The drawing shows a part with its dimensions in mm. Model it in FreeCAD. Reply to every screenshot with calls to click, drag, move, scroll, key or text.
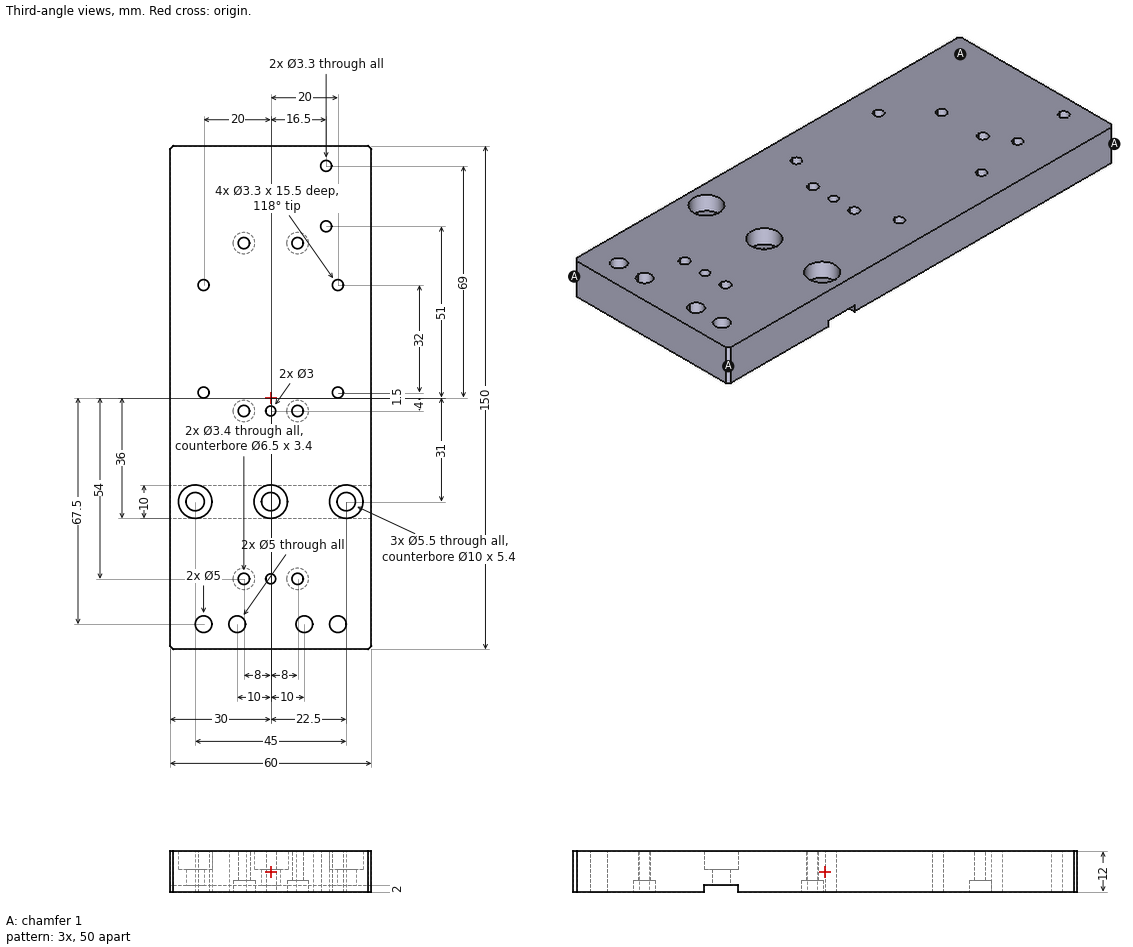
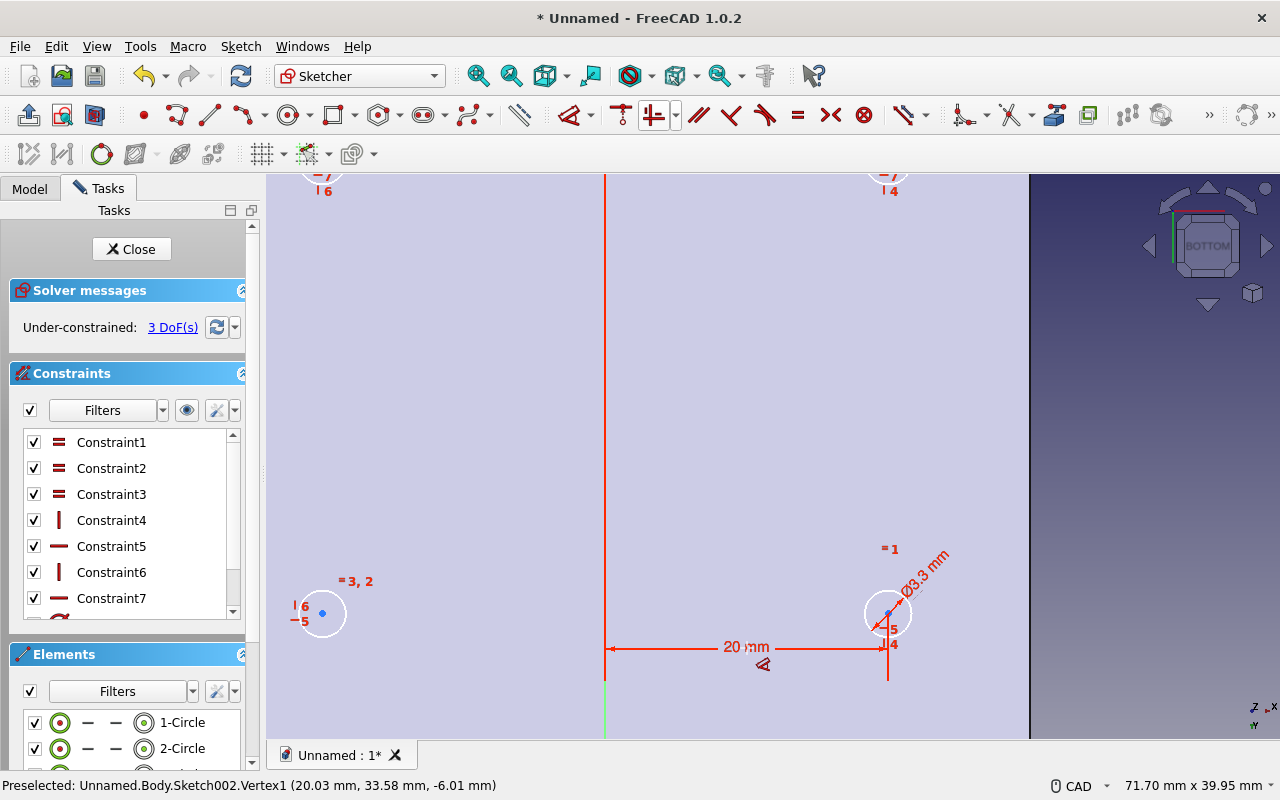
click(323, 614)
click(464, 648)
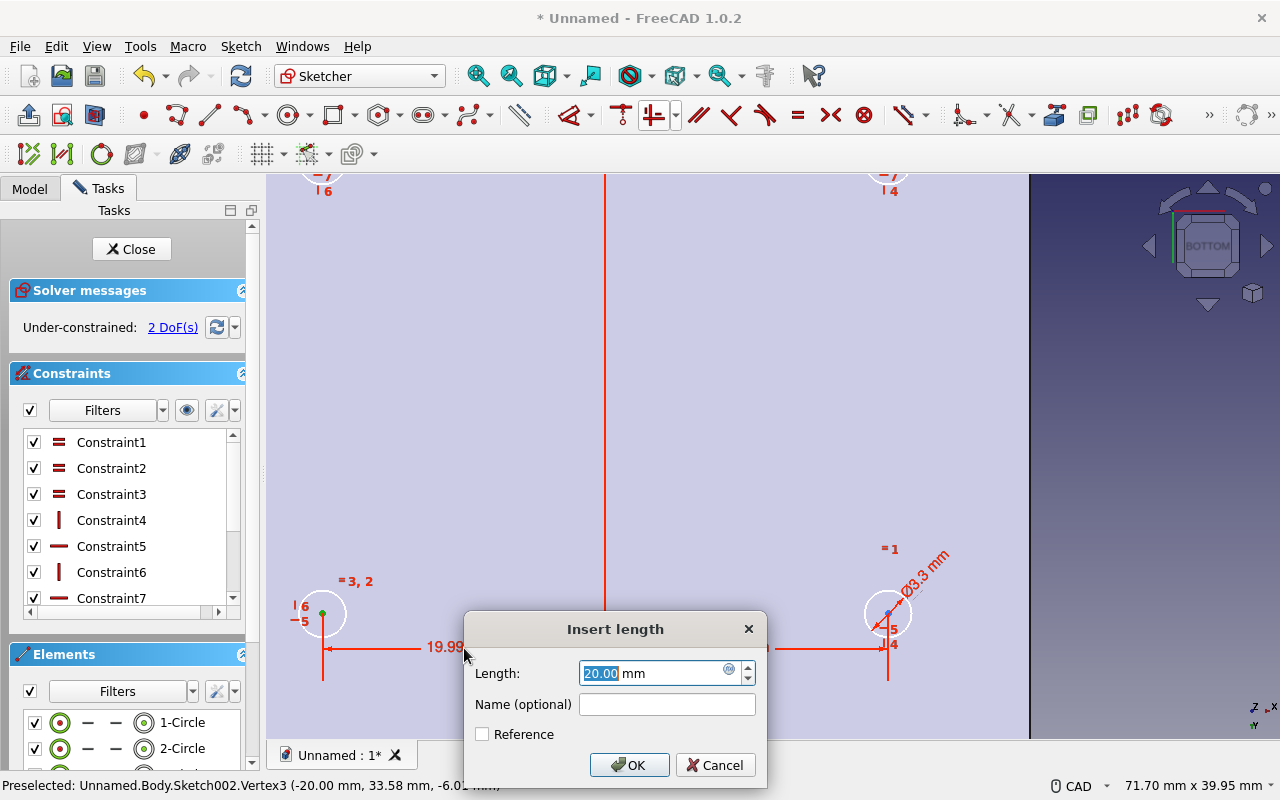
text(20)
key(Return)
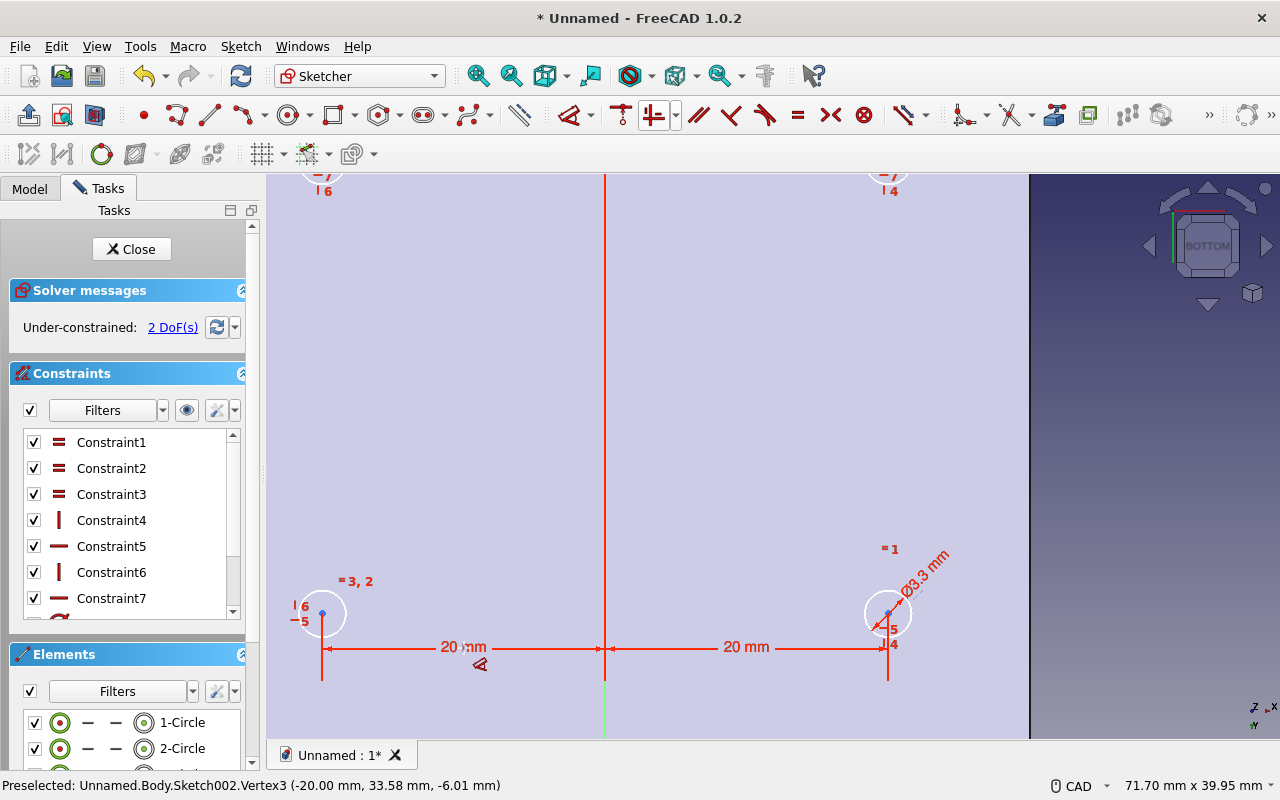
scroll(906, 599, down, 2)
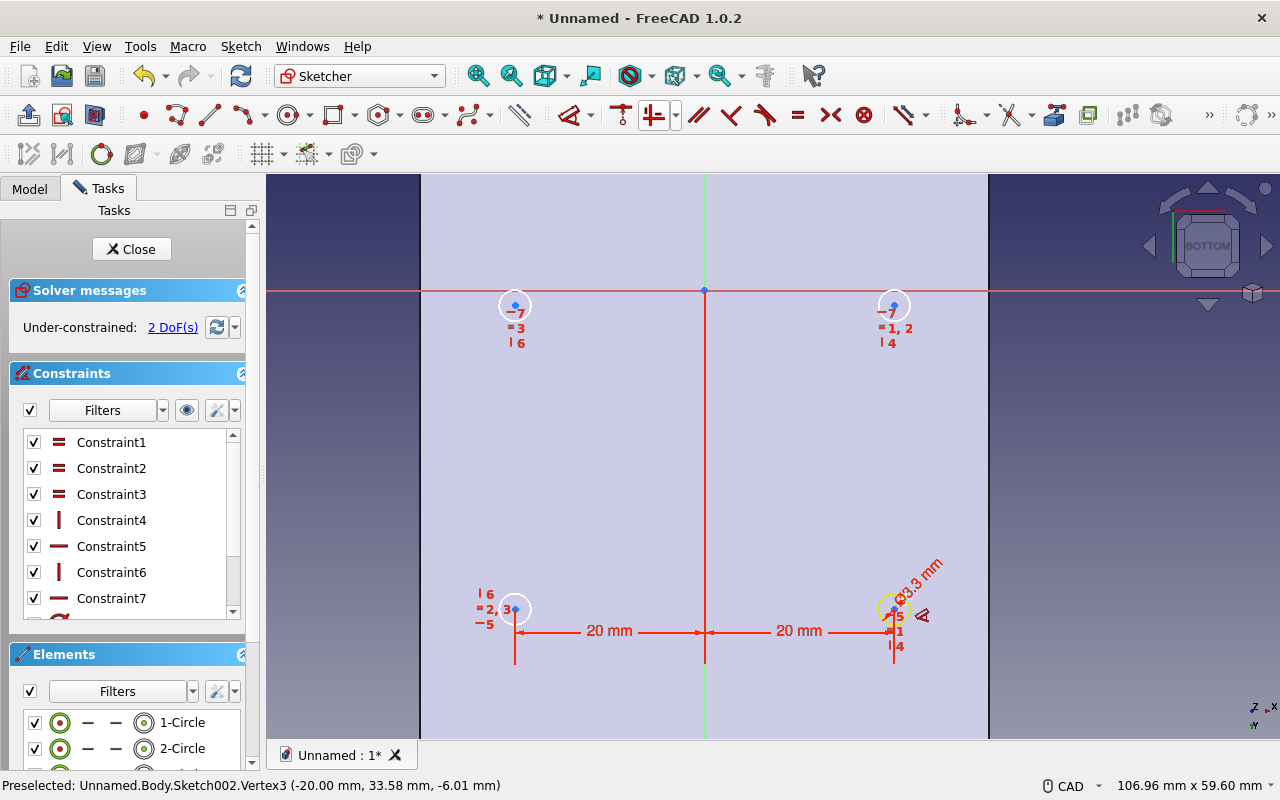
scroll(894, 306, up, 6)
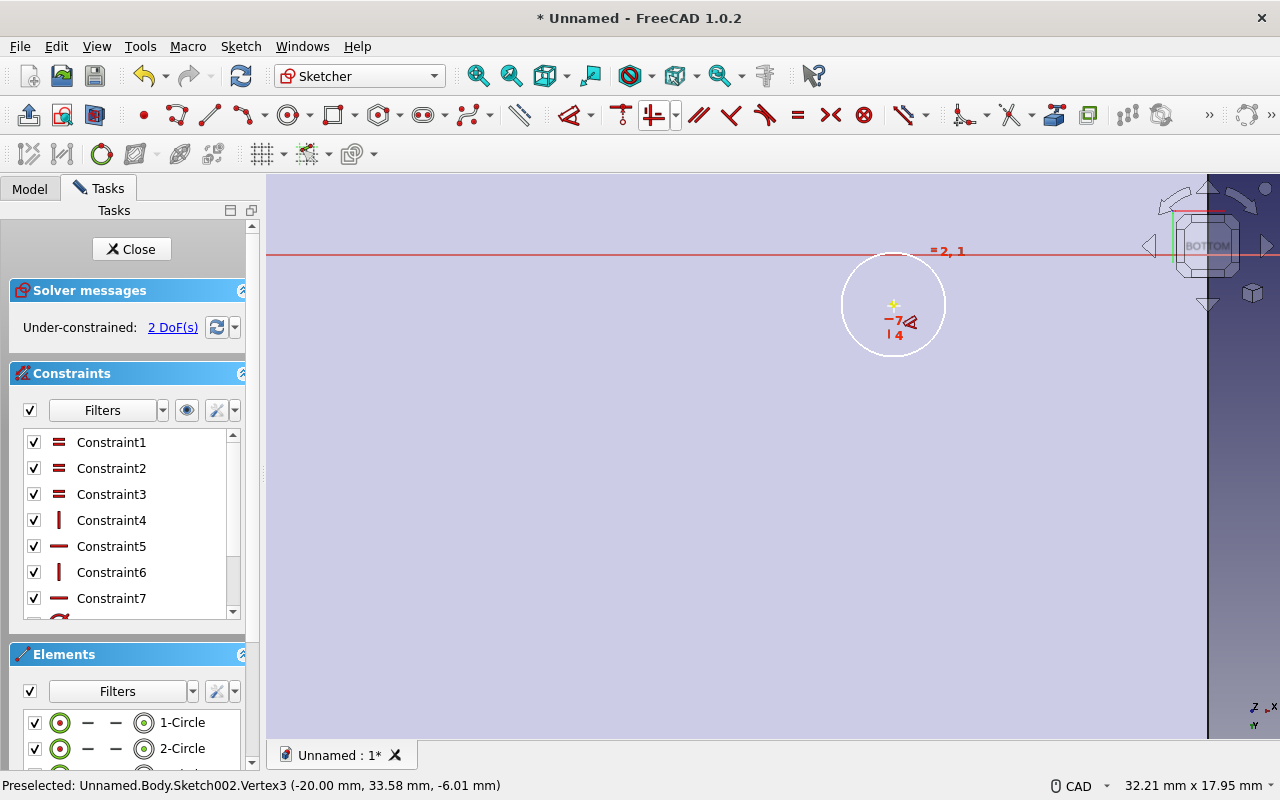
click(893, 305)
click(927, 291)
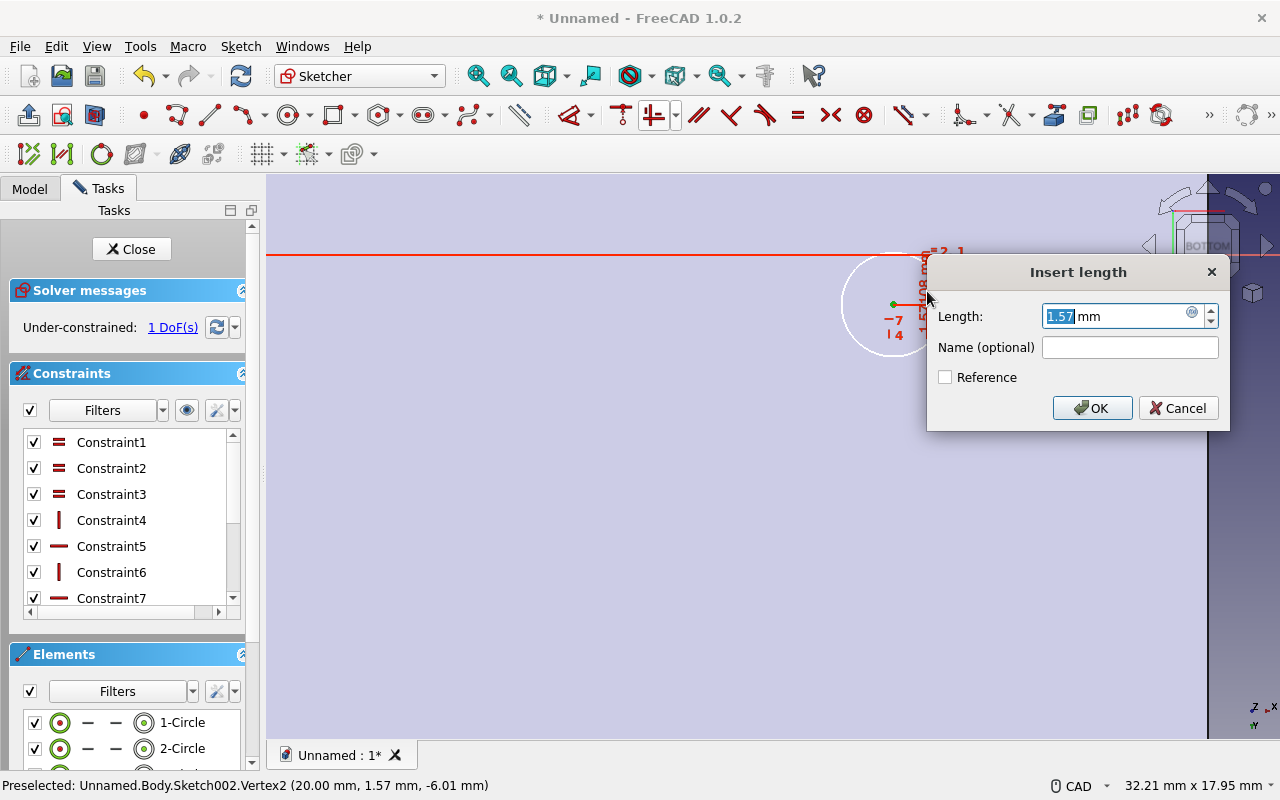
text(1.5)
key(Return)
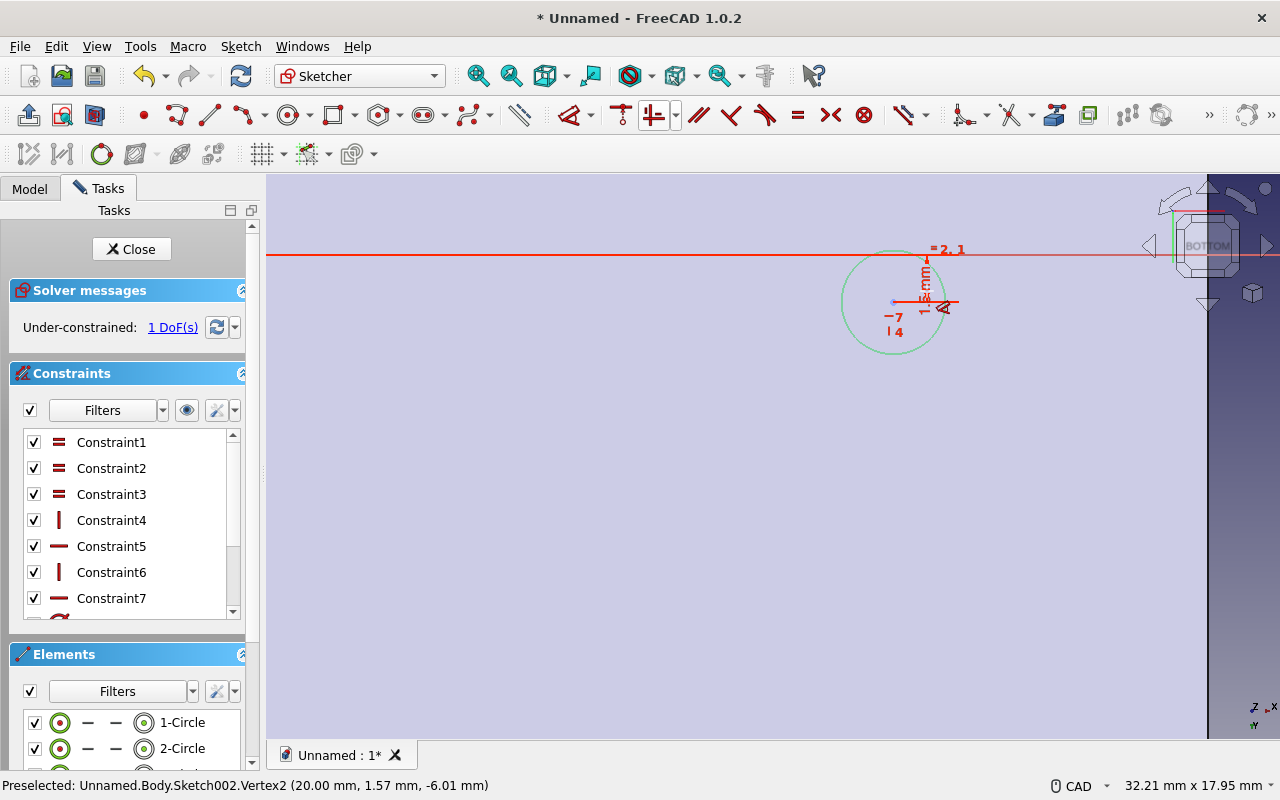
scroll(894, 306, down, 6)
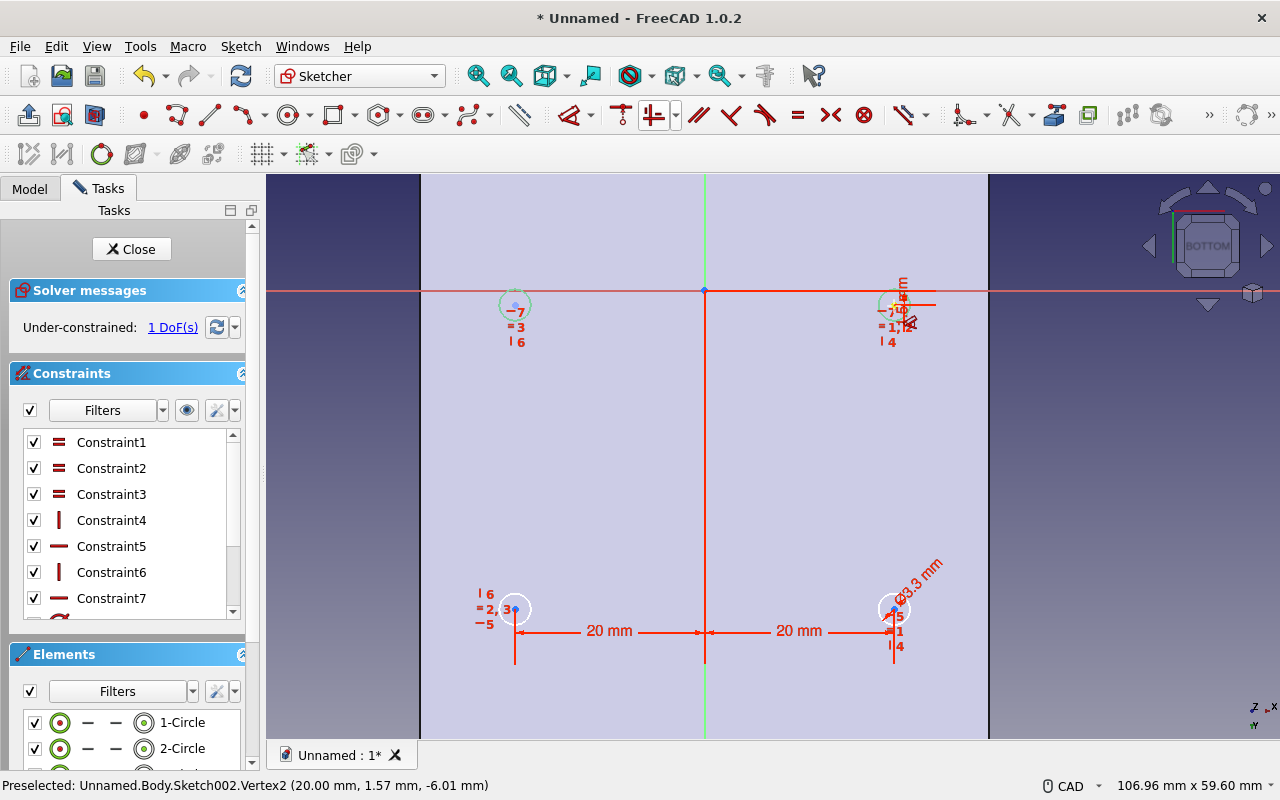
click(894, 609)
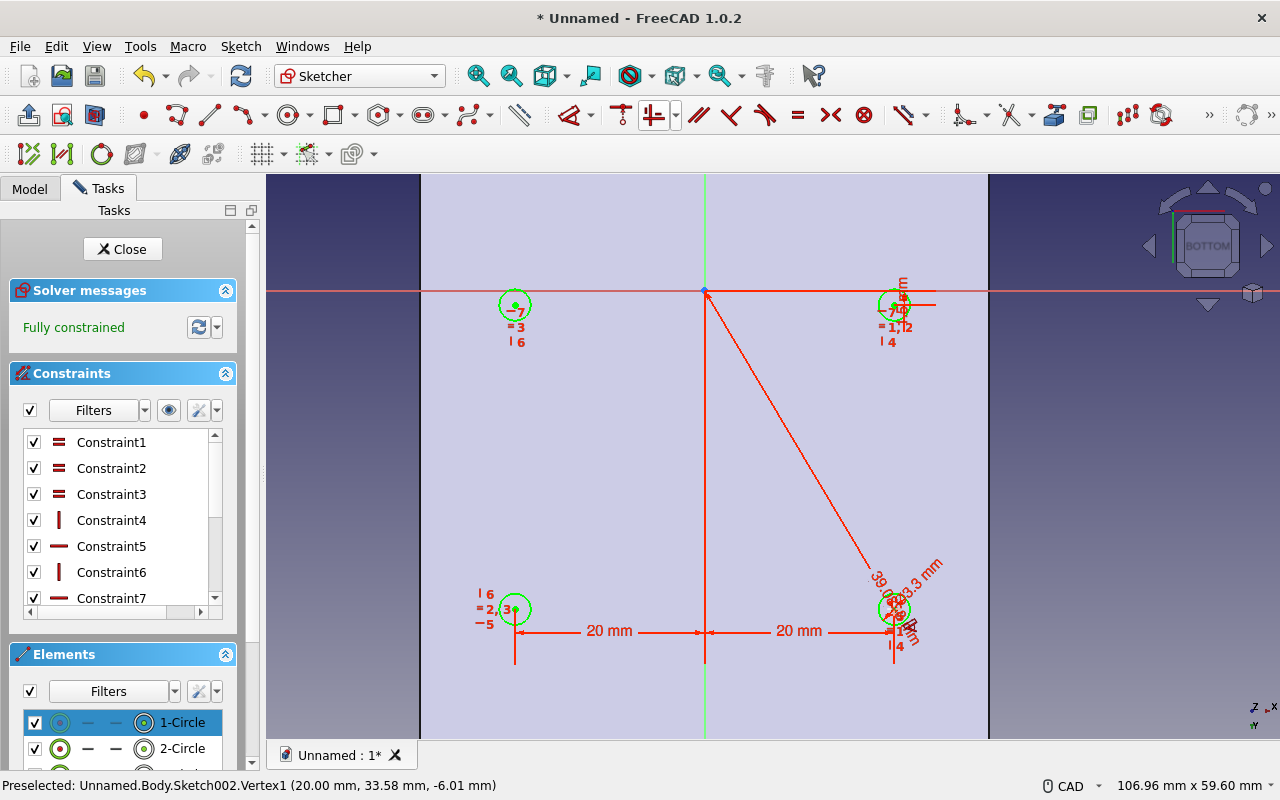
click(894, 305)
click(928, 457)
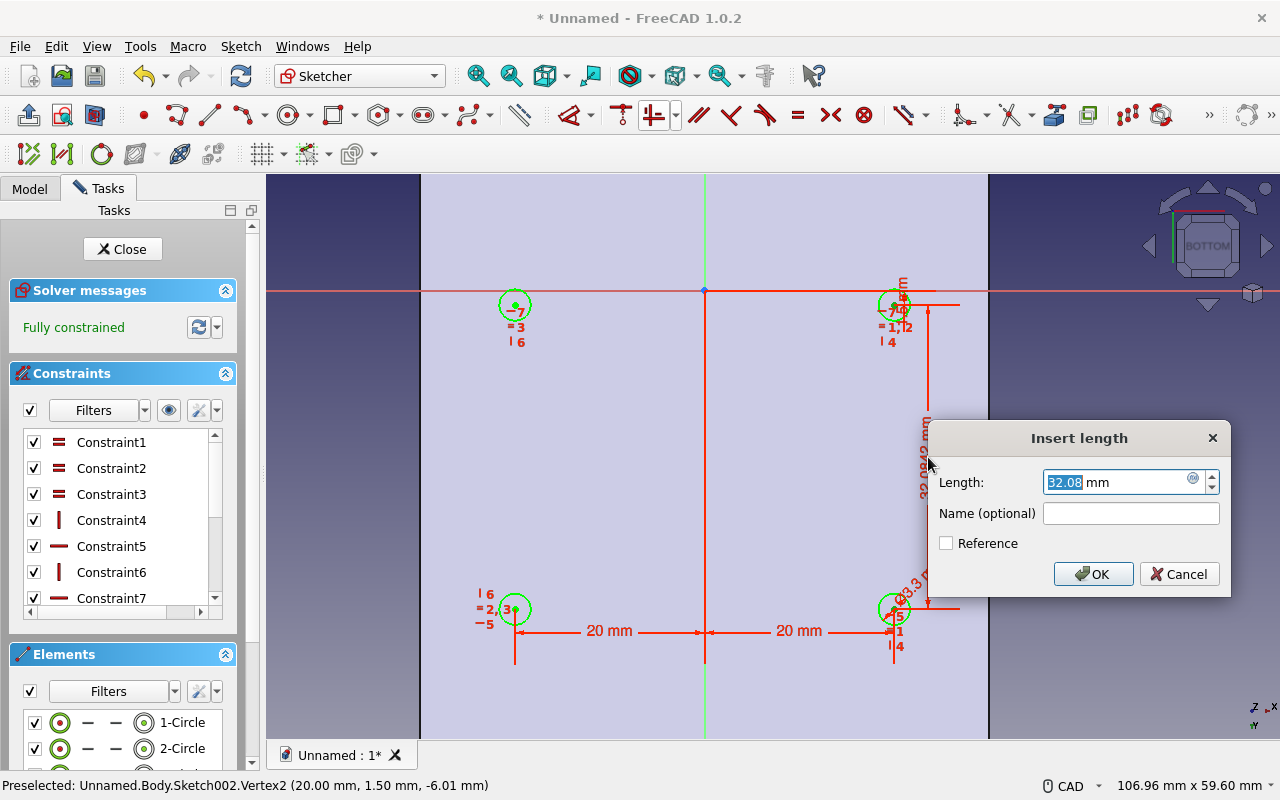
text(32)
key(Return)
key(Escape)